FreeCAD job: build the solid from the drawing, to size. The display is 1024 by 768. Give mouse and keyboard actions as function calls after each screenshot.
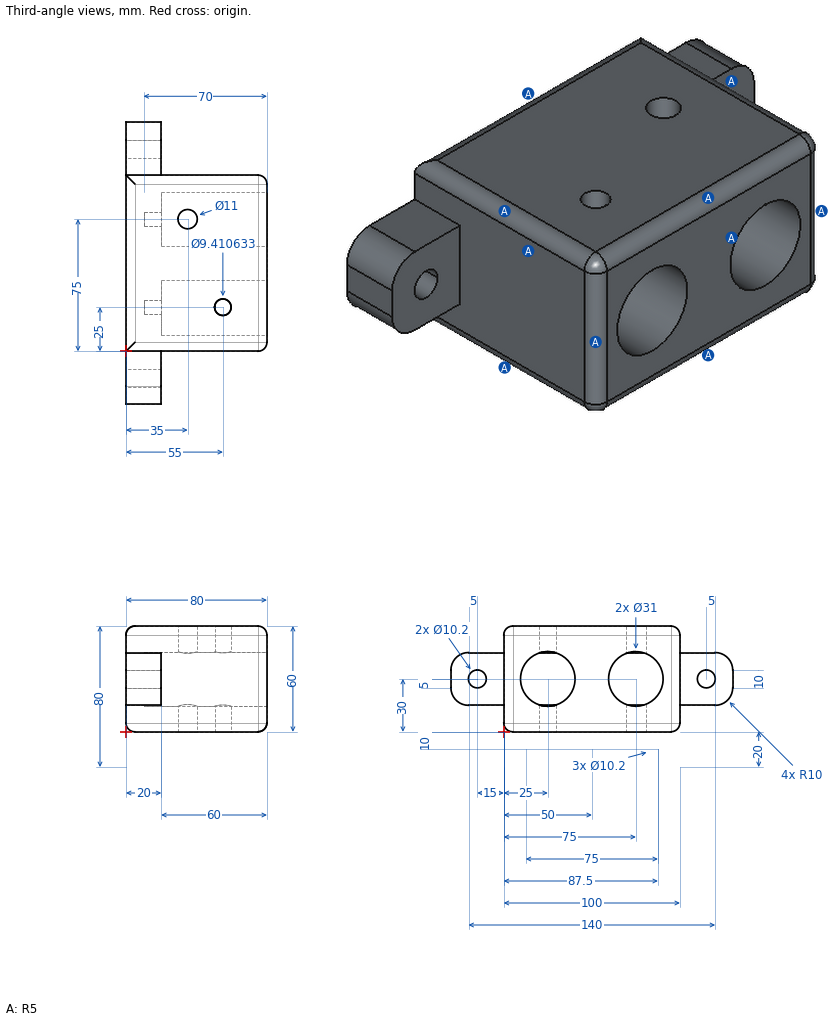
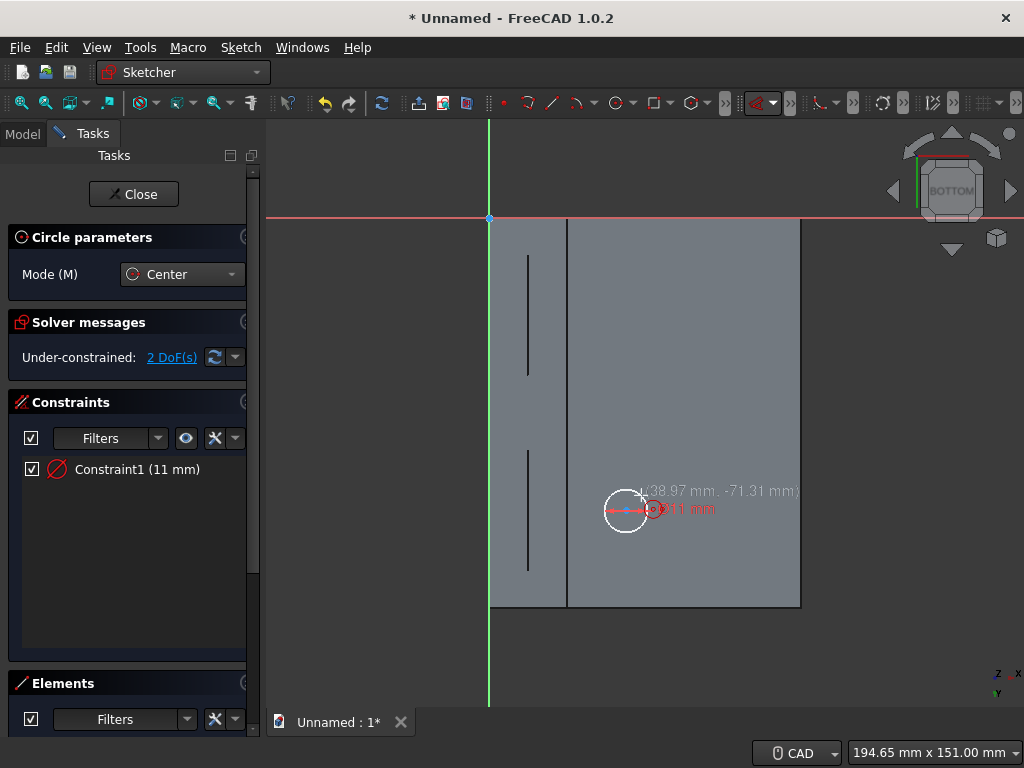
scroll(703, 316, up, 2)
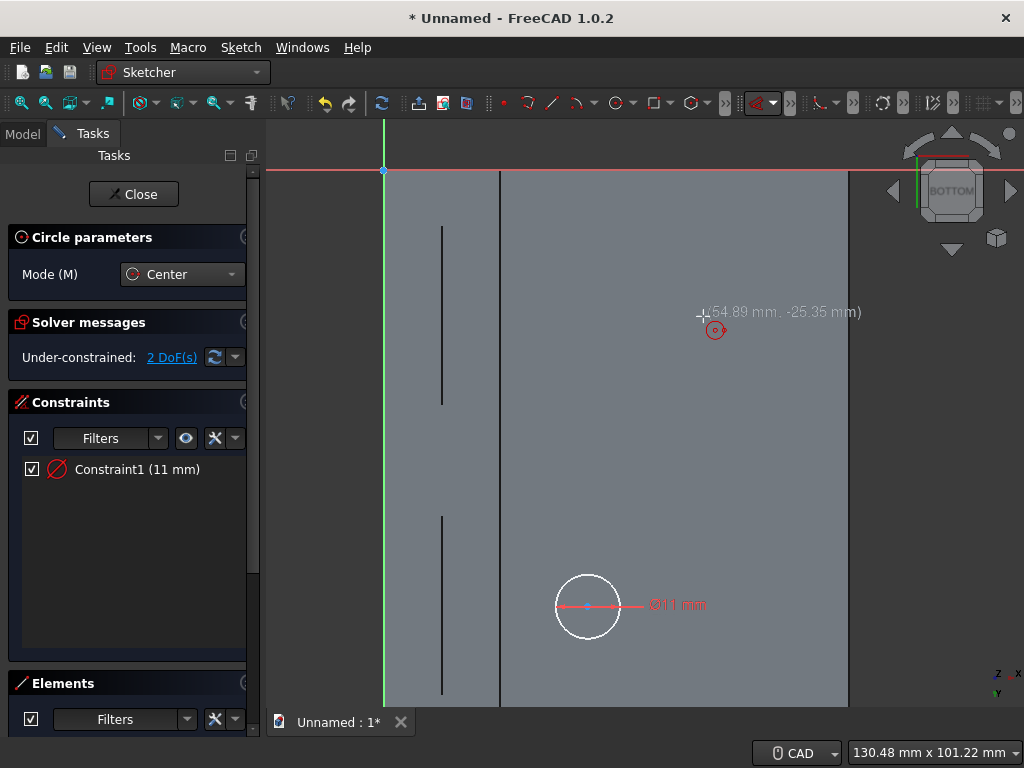
click(703, 315)
move(723, 296)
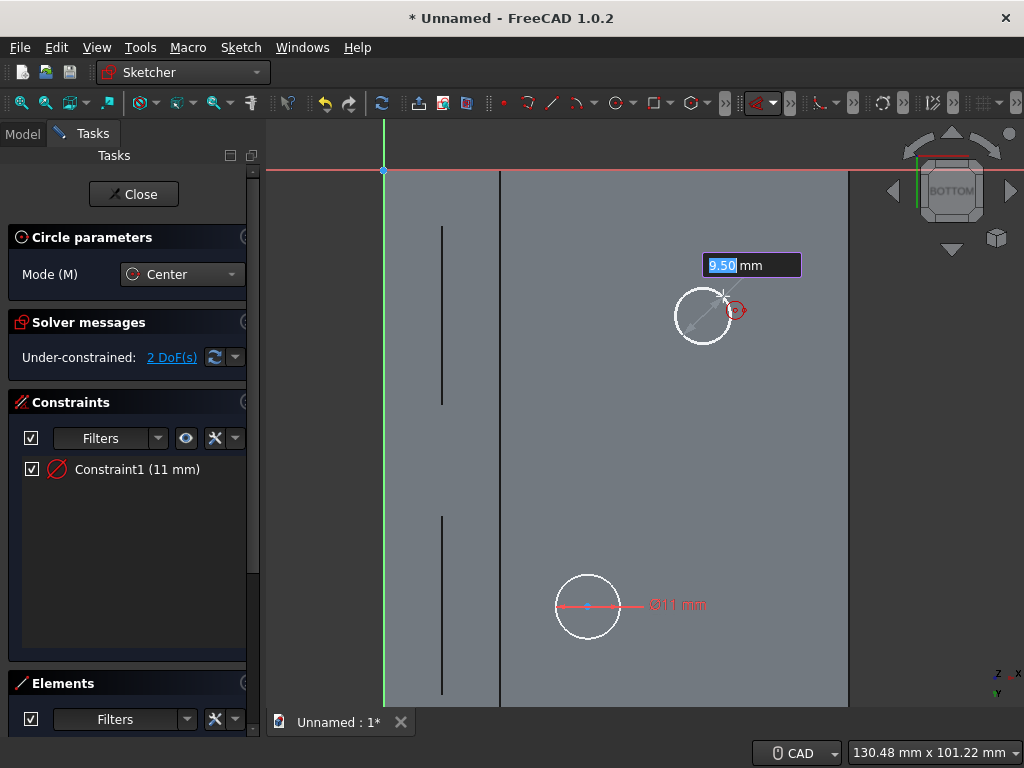
text(9.410633)
key(Return)
key(Escape)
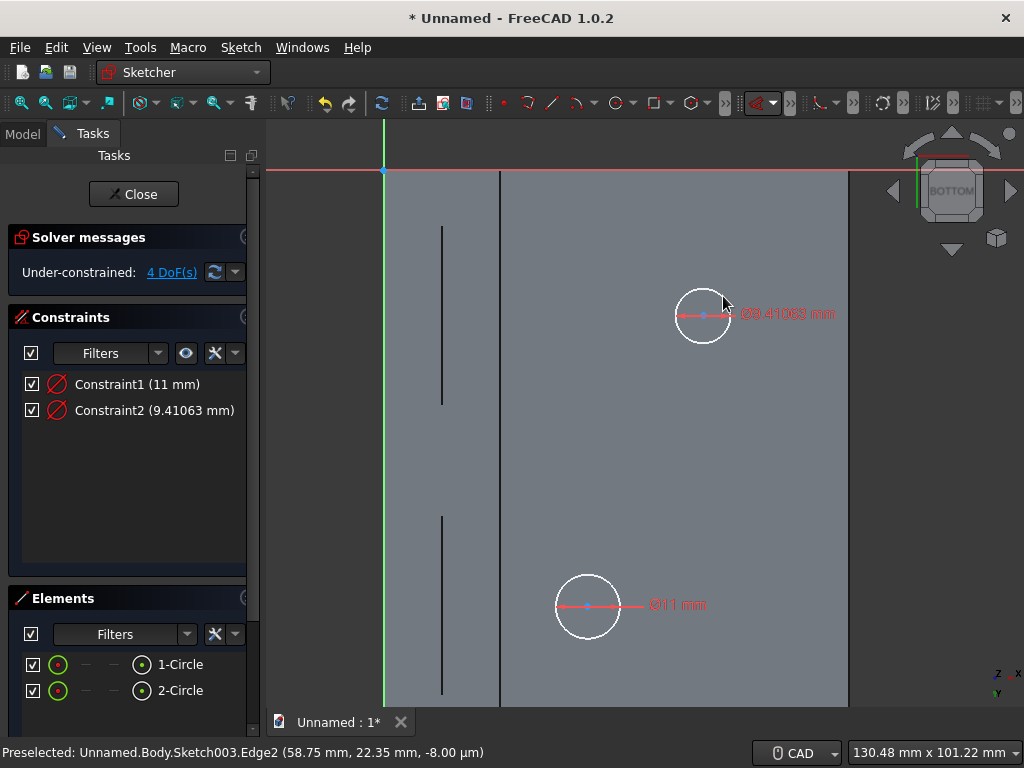
click(588, 607)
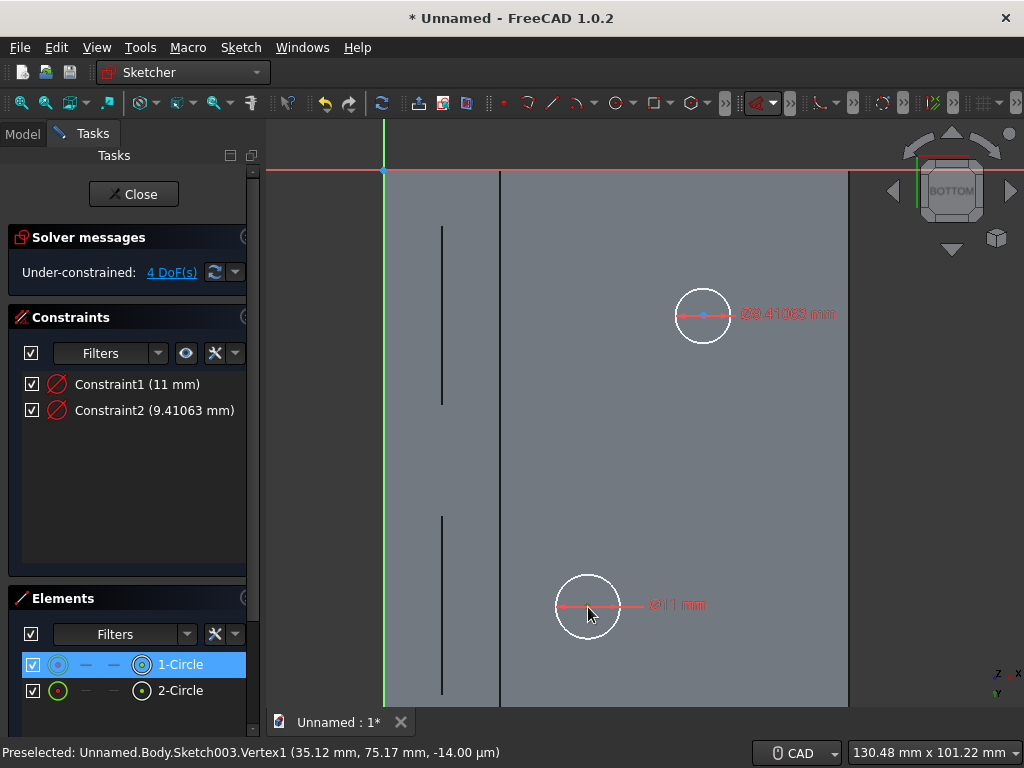
key(l)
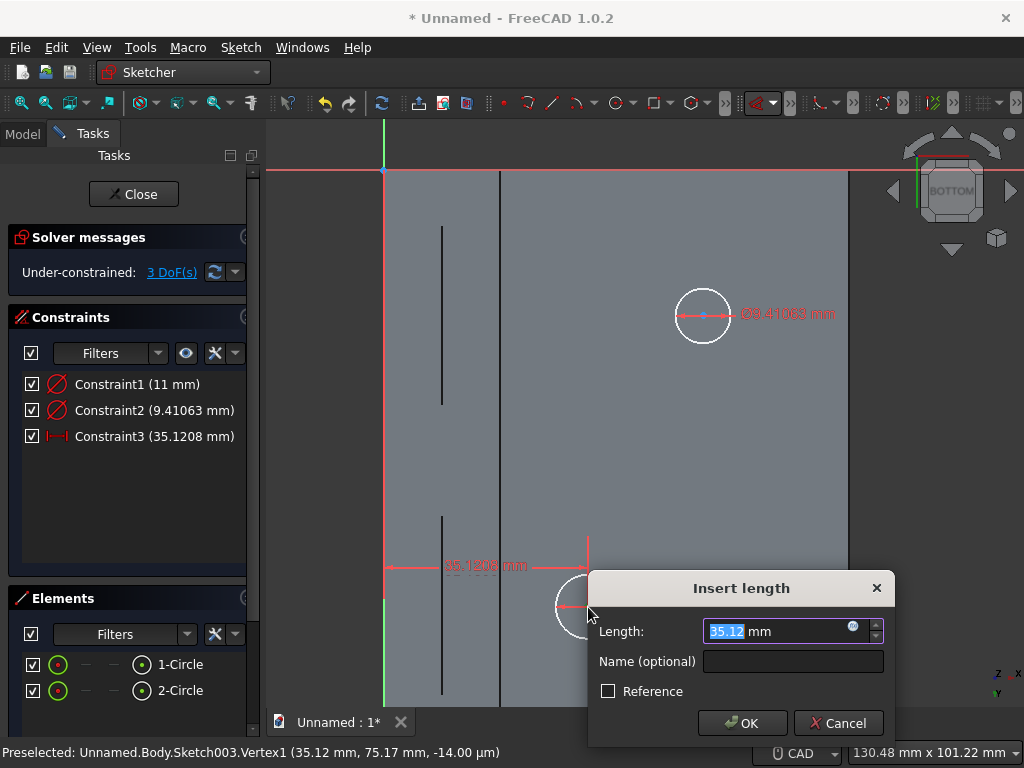
text(35)
key(Return)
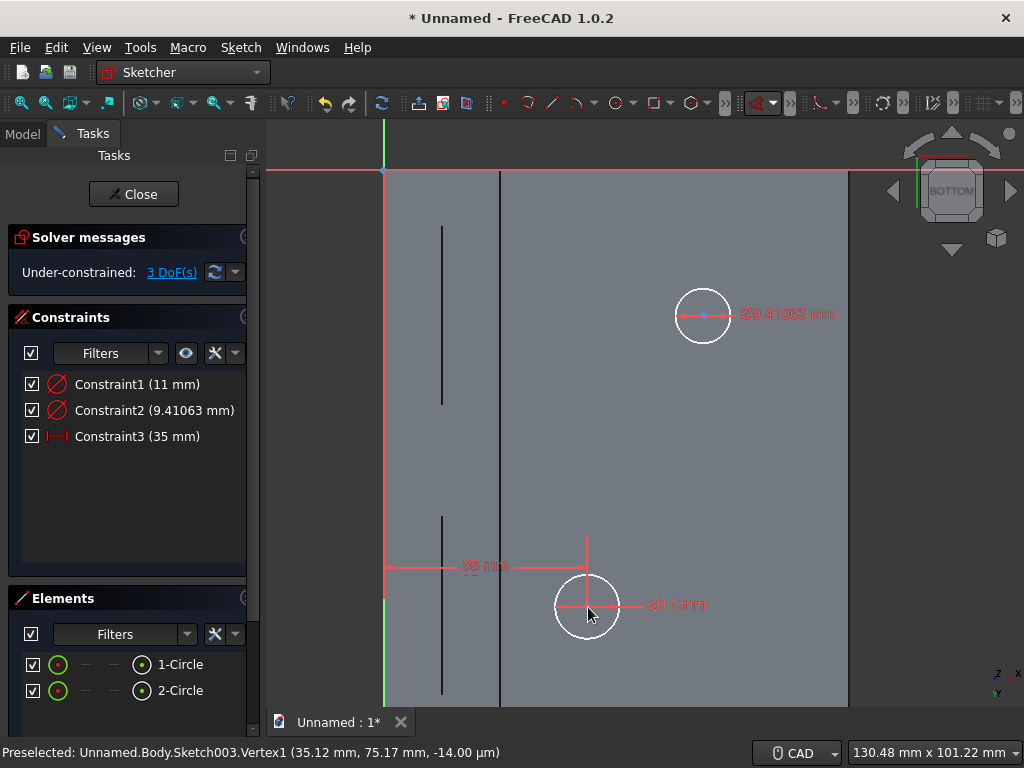
click(587, 607)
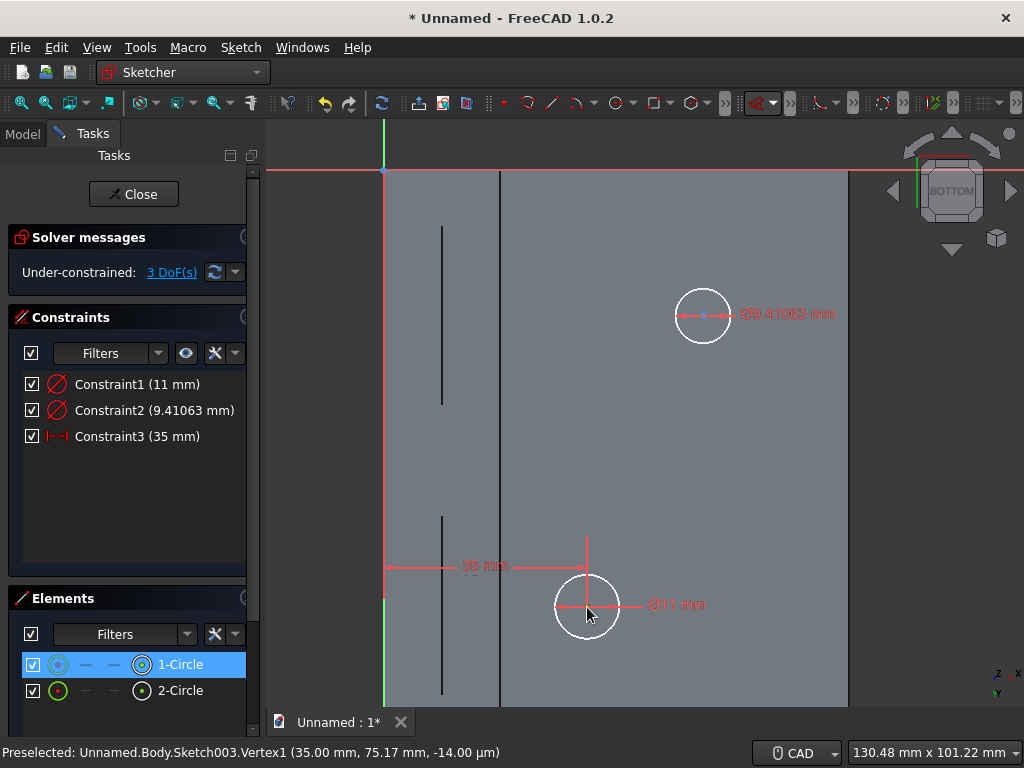
key(i)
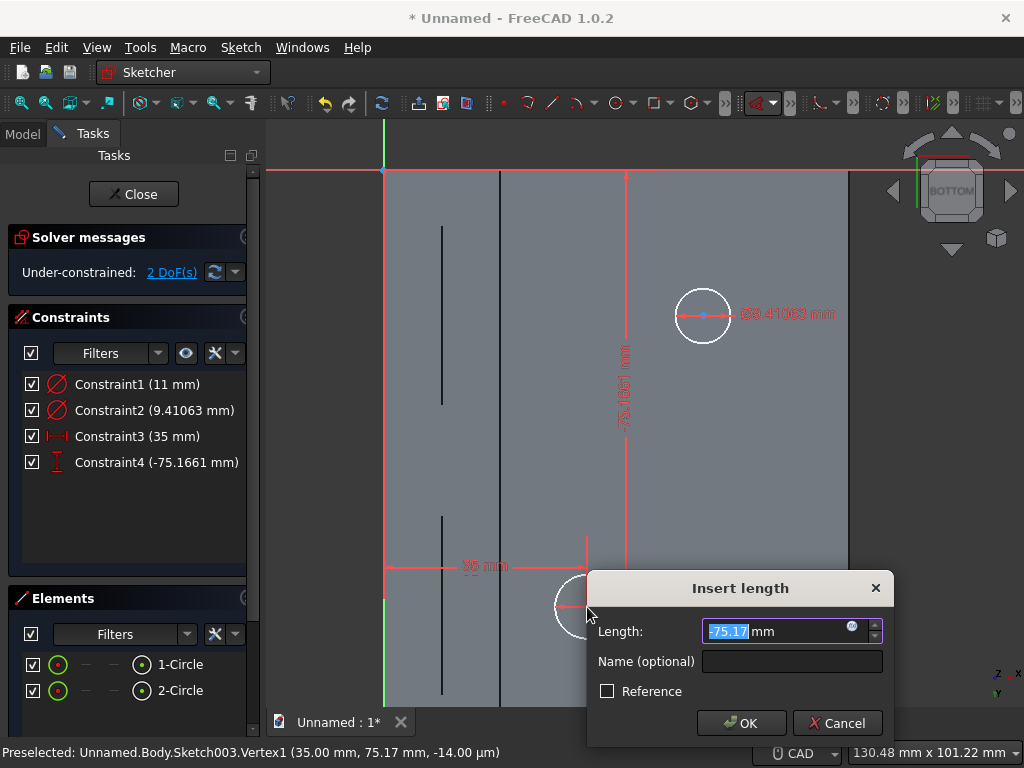
text(-75)
key(Return)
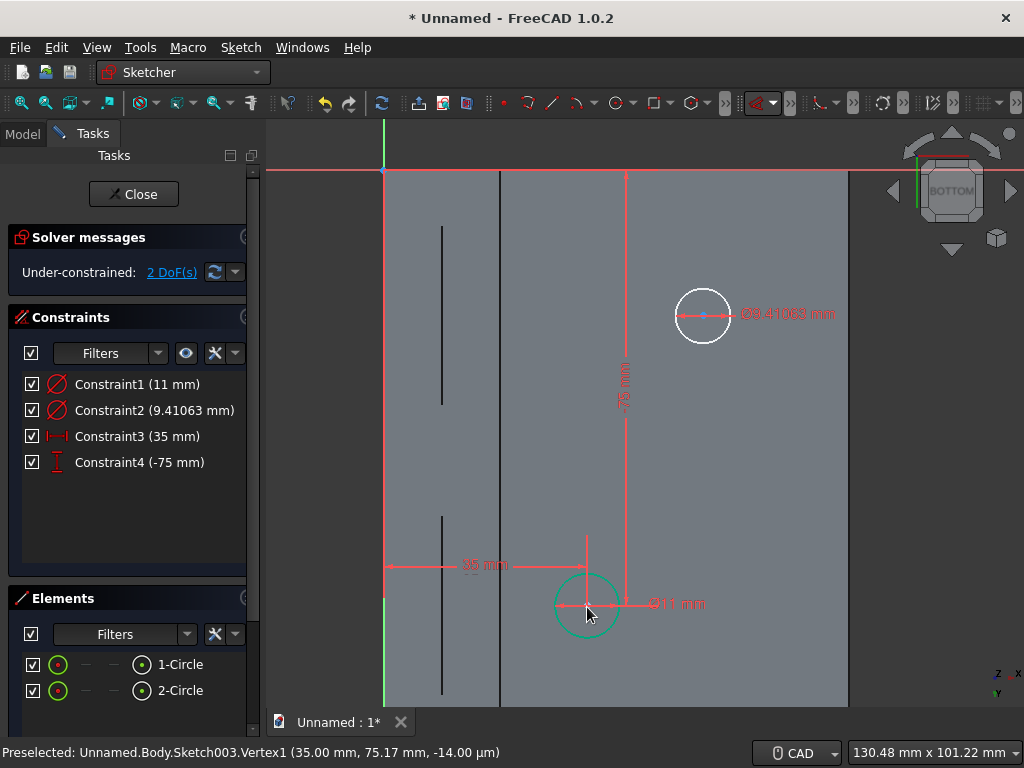
click(703, 316)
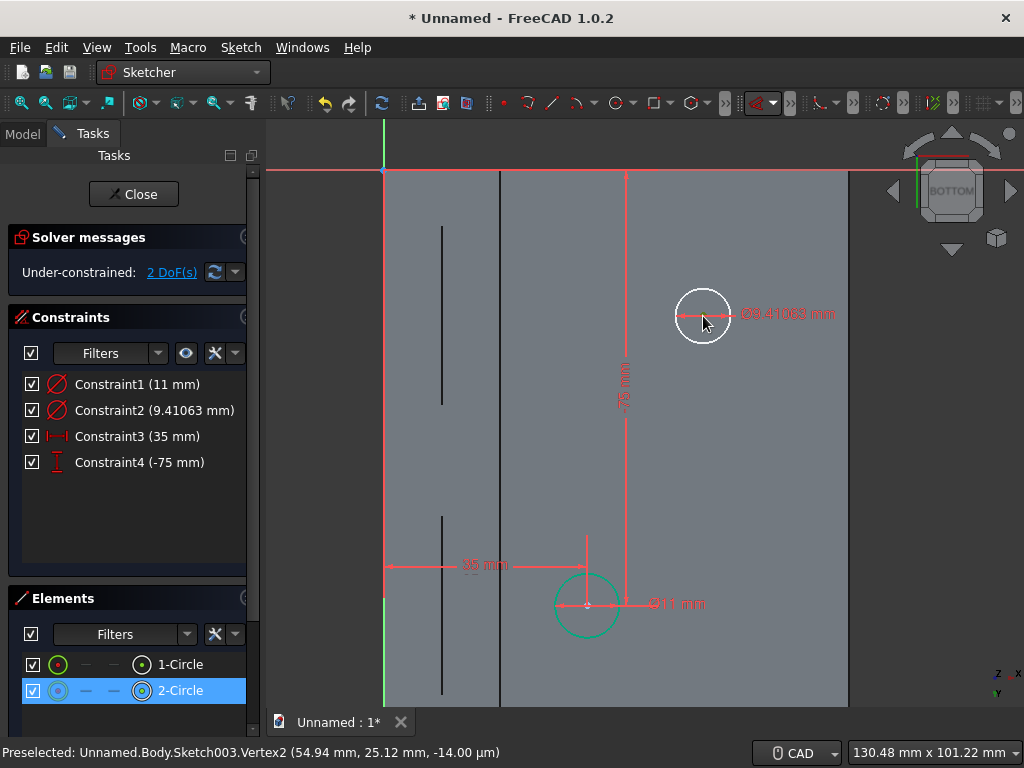
key(l)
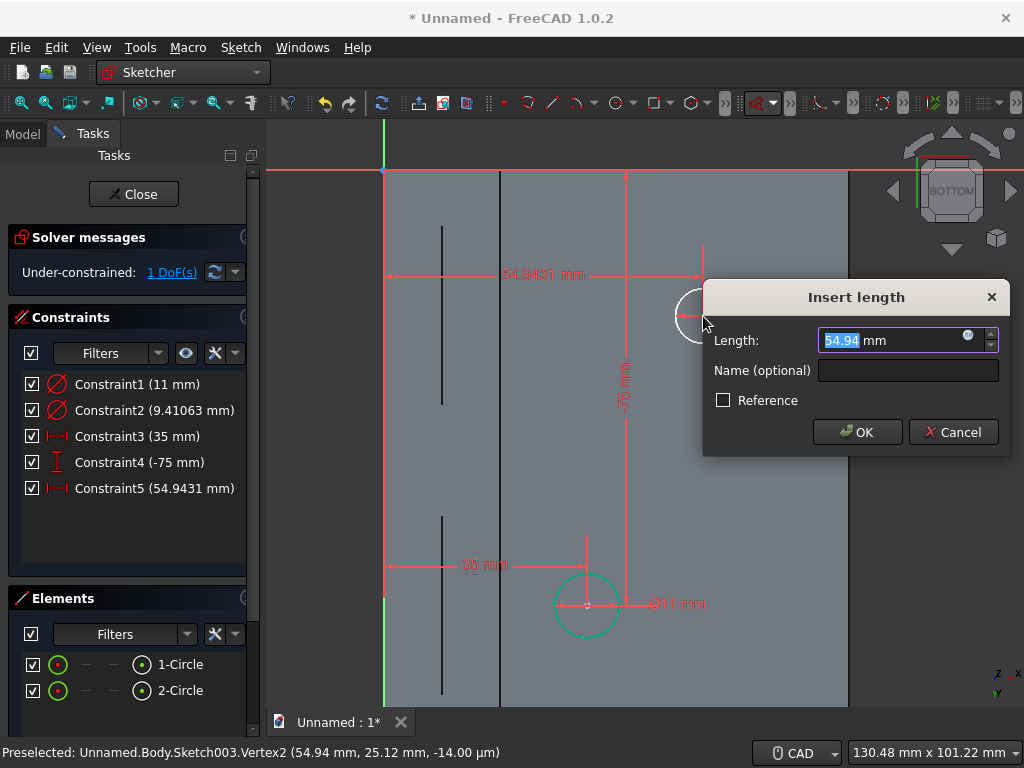
text(55)
key(Return)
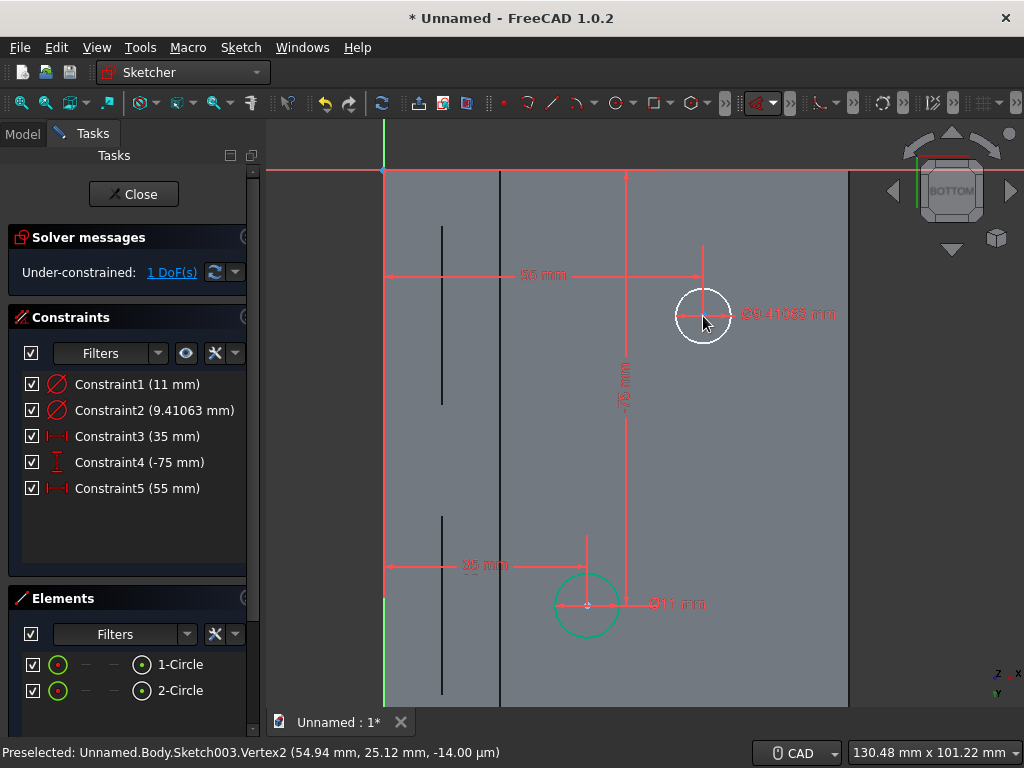
click(703, 316)